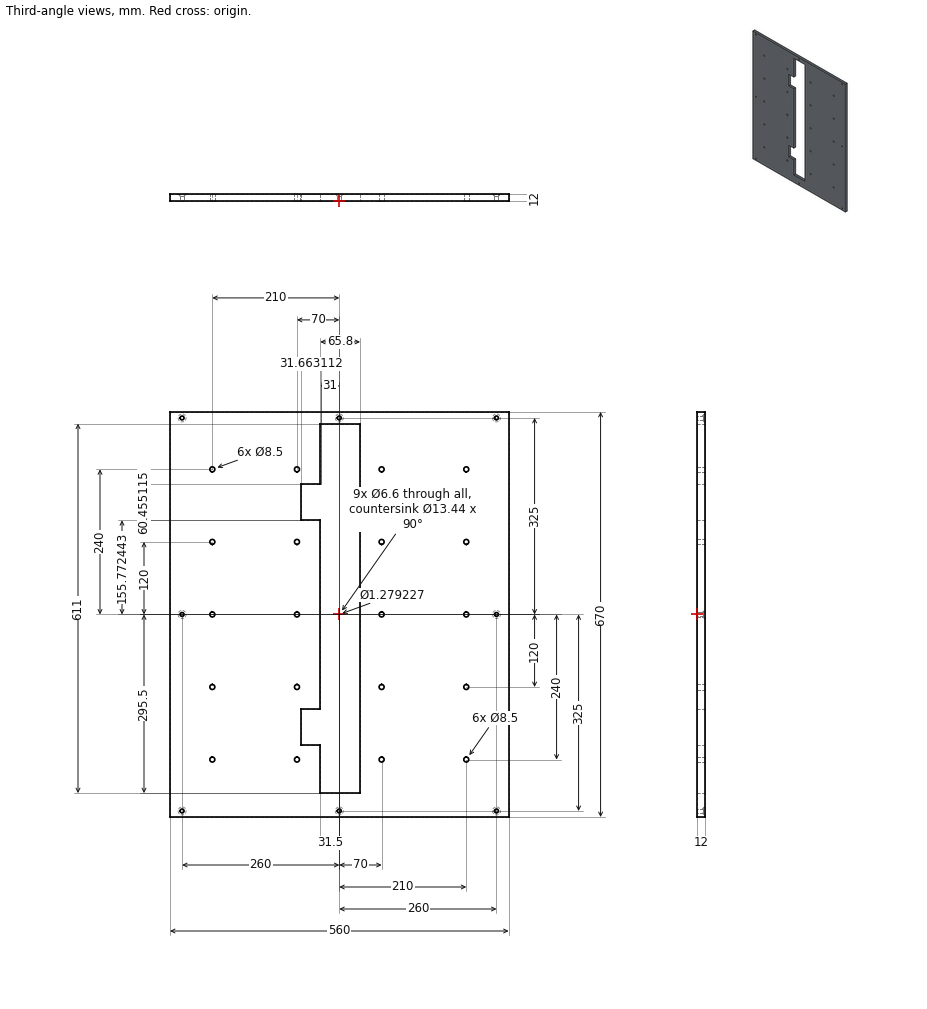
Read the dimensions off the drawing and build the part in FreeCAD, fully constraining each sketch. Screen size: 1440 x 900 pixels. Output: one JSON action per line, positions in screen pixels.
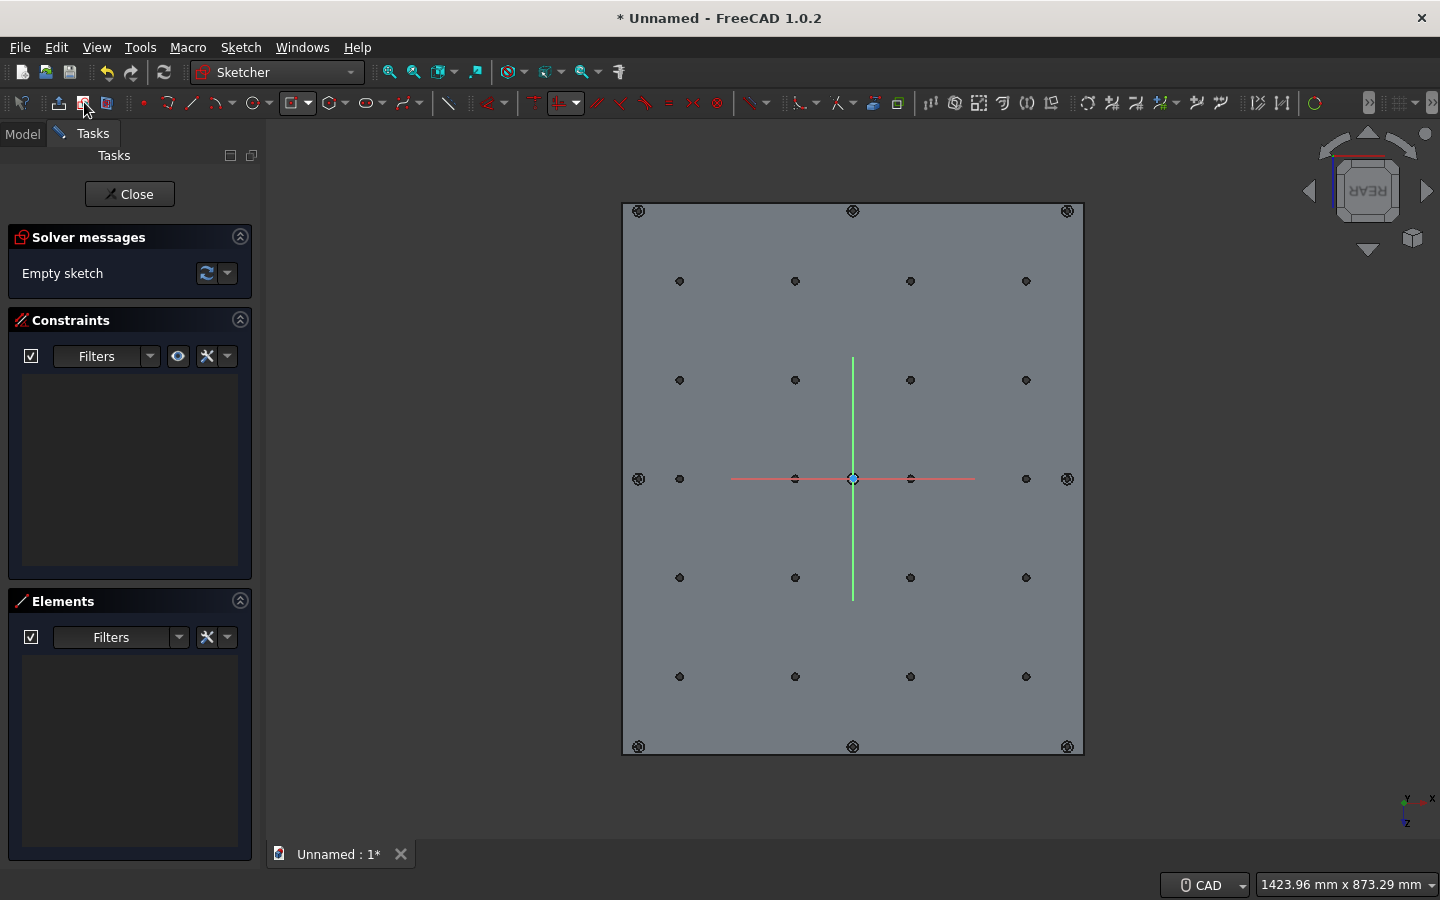
{"action": "left_click", "coordinate": [310, 104]}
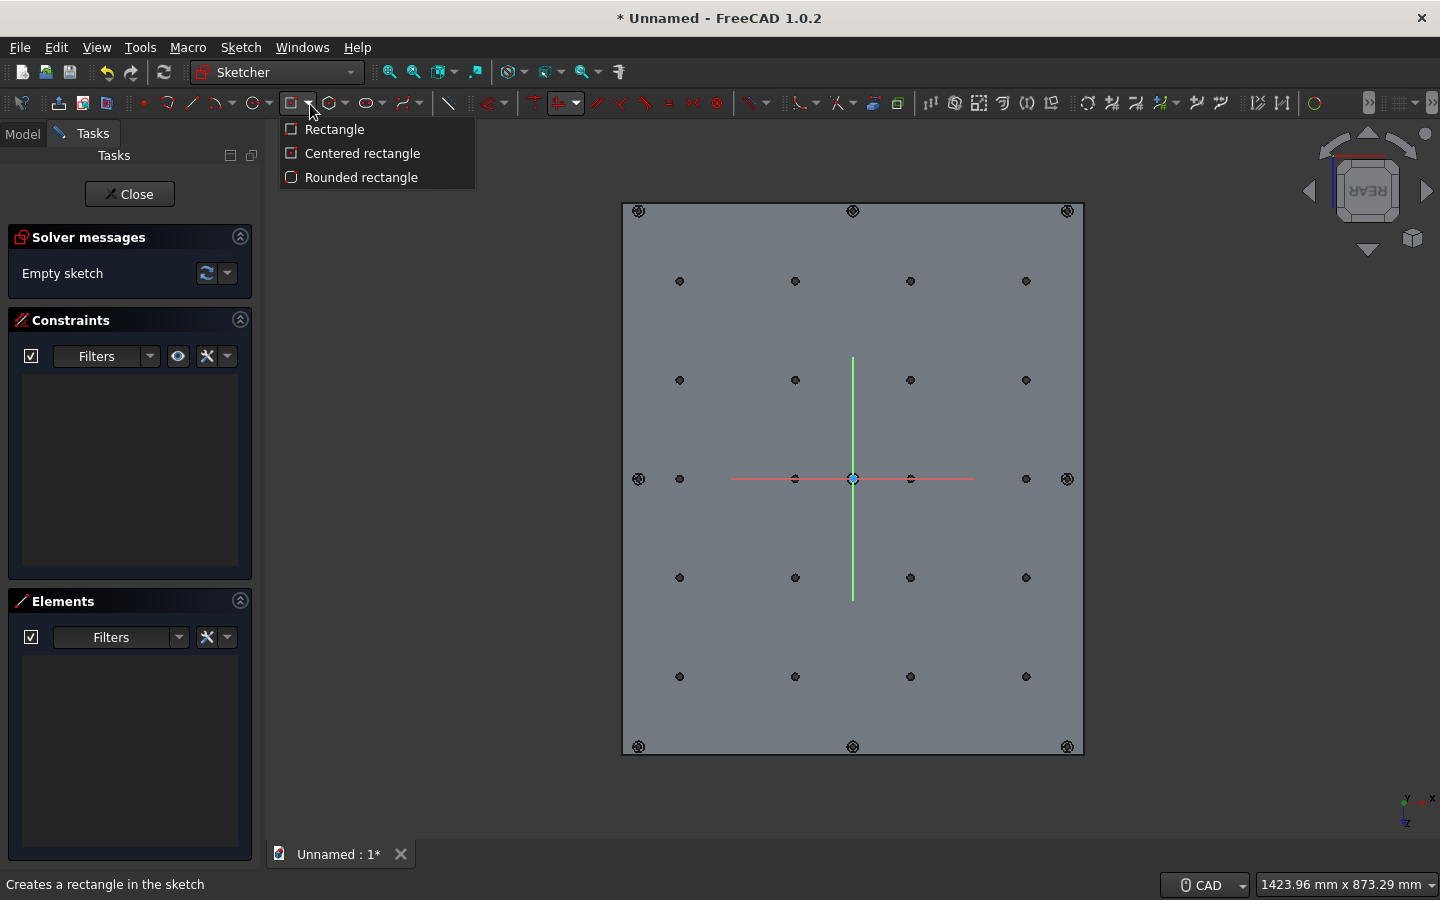
{"action": "left_click", "coordinate": [378, 129]}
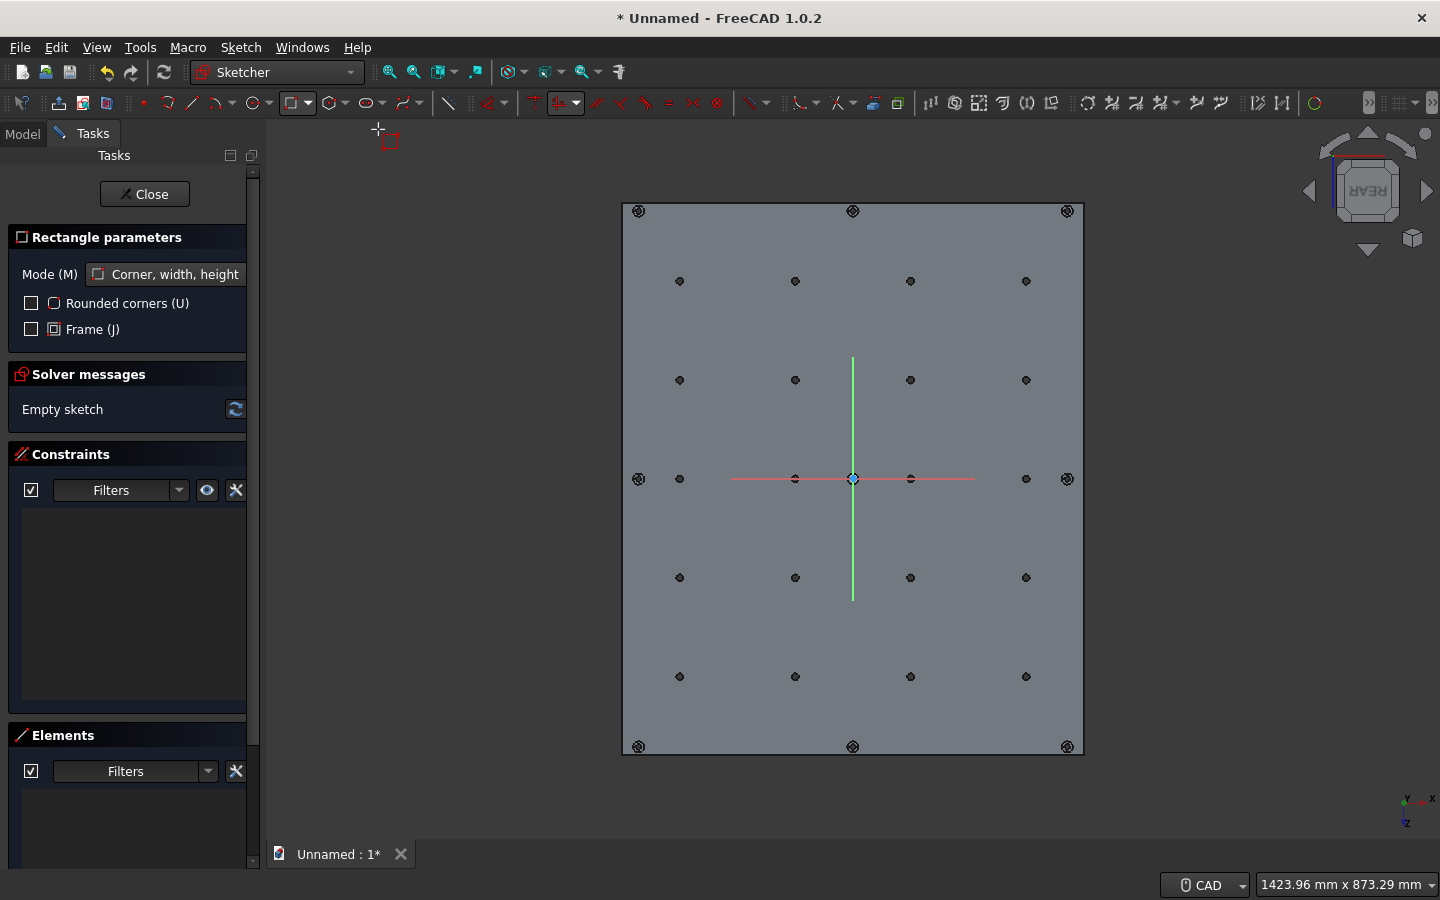
{"action": "left_click", "coordinate": [827, 235]}
{"action": "left_click", "coordinate": [881, 739]}
{"action": "key", "text": "Escape"}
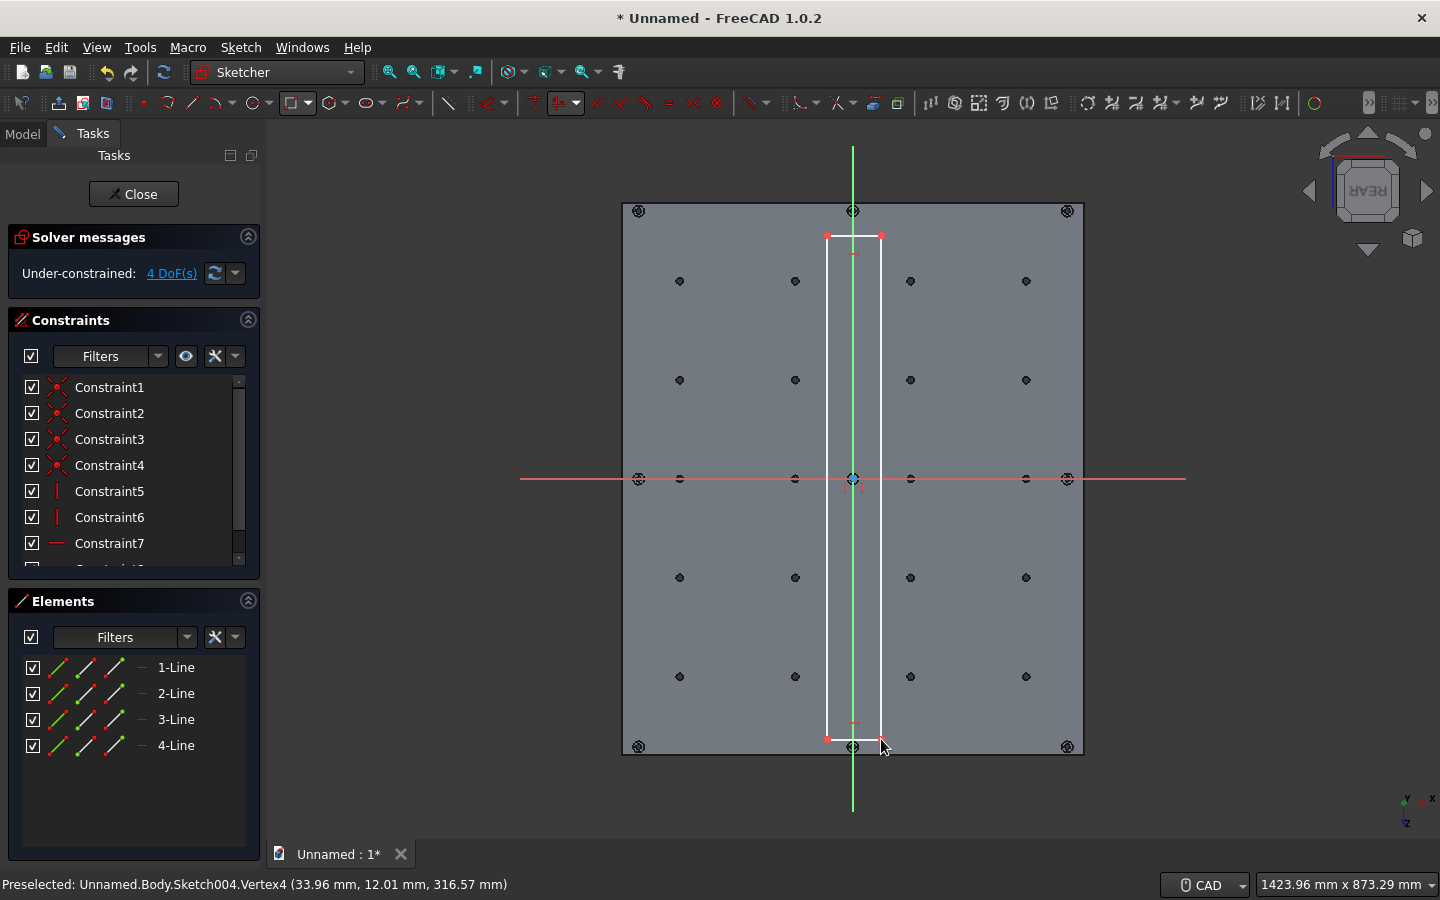
{"action": "left_click", "coordinate": [488, 104]}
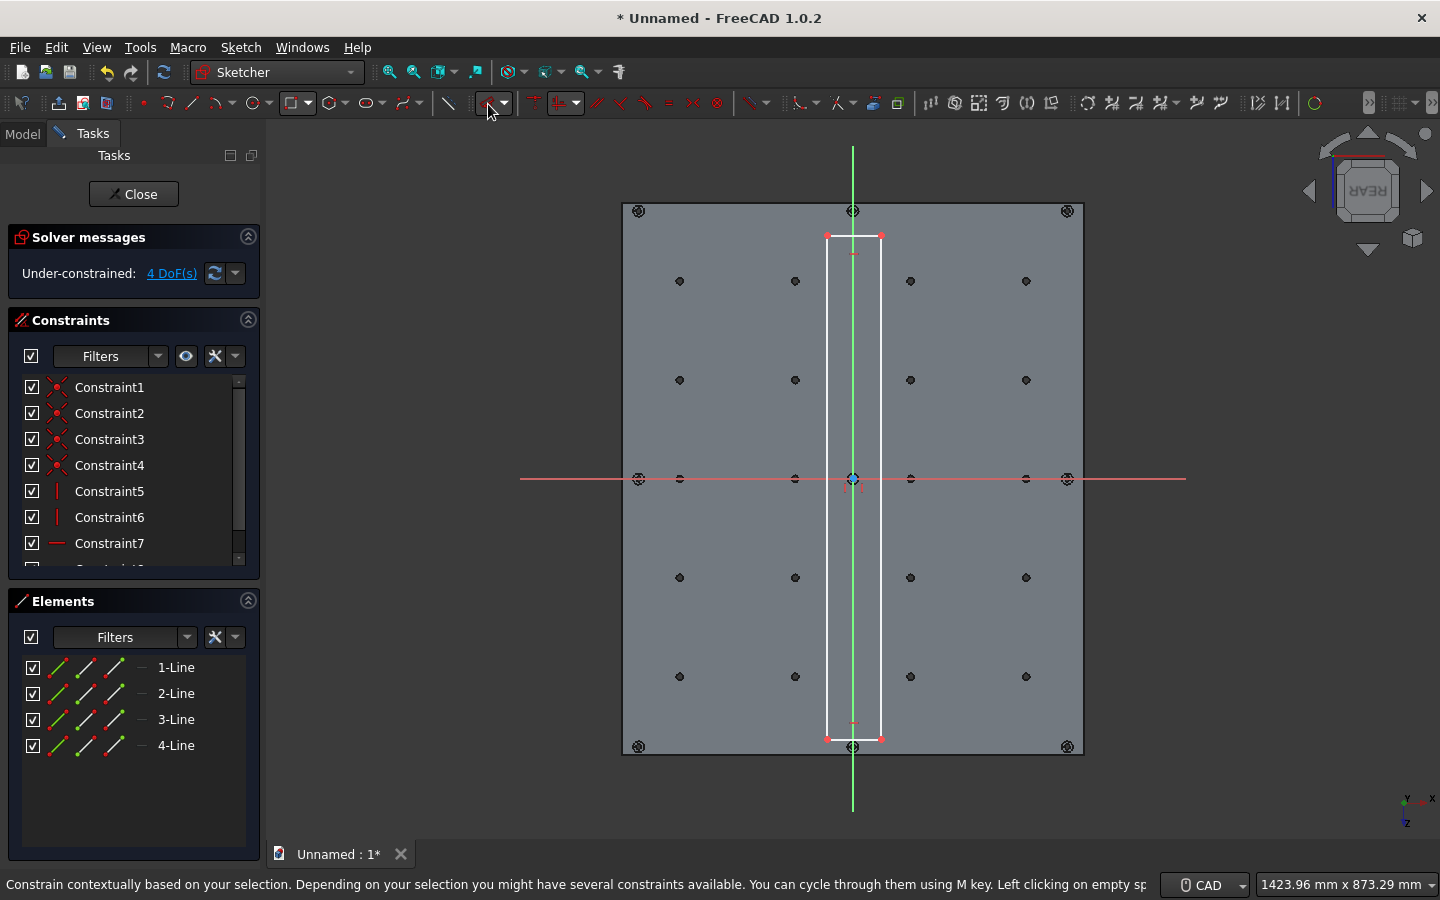
{"action": "left_click", "coordinate": [827, 387]}
{"action": "left_click", "coordinate": [793, 372]}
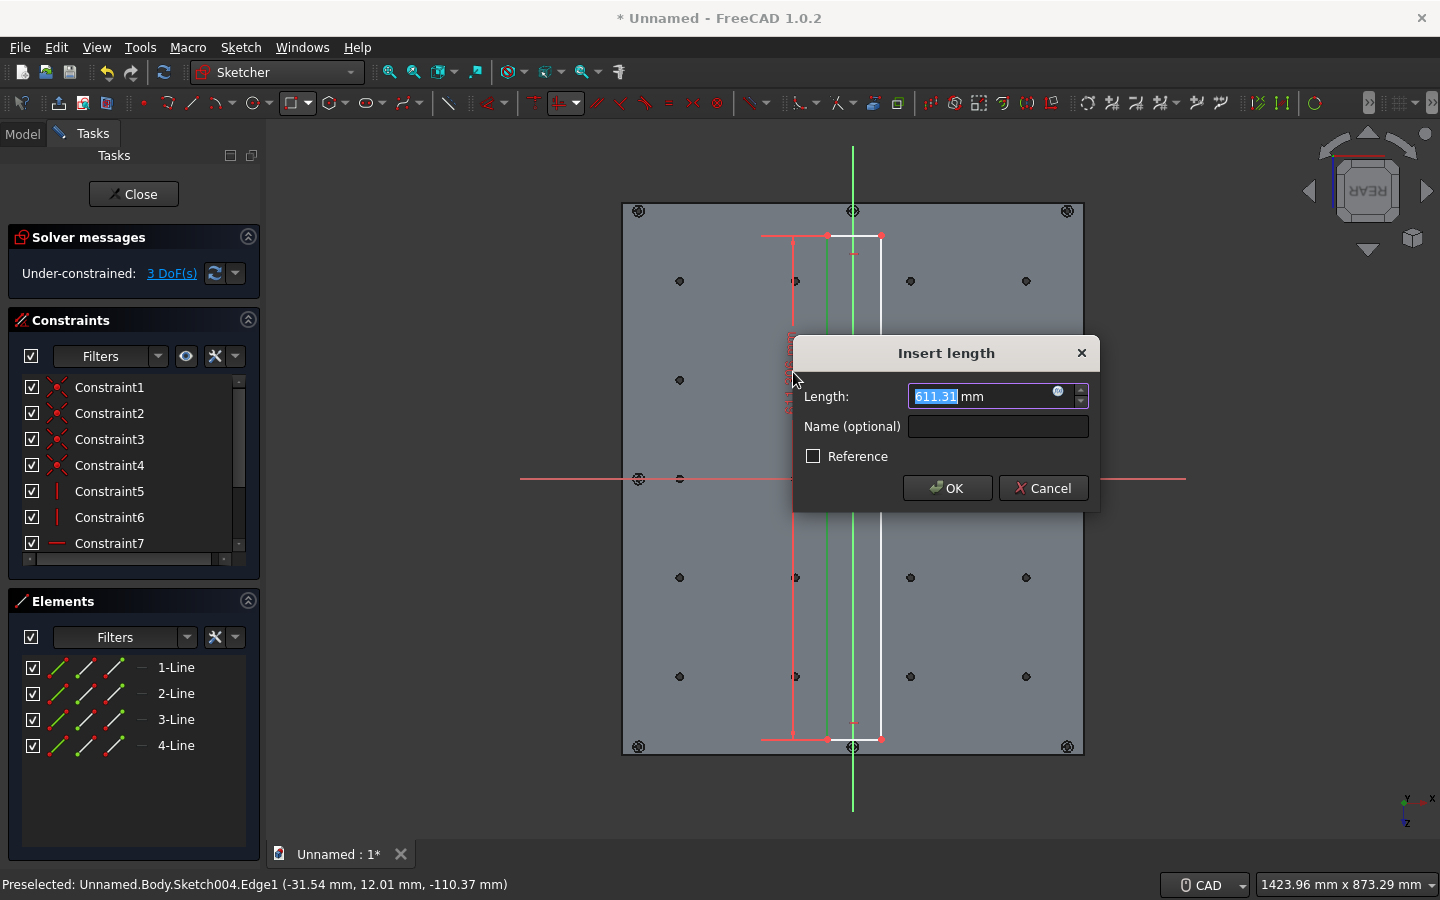
{"action": "type", "text": "611"}
{"action": "key", "text": "Return"}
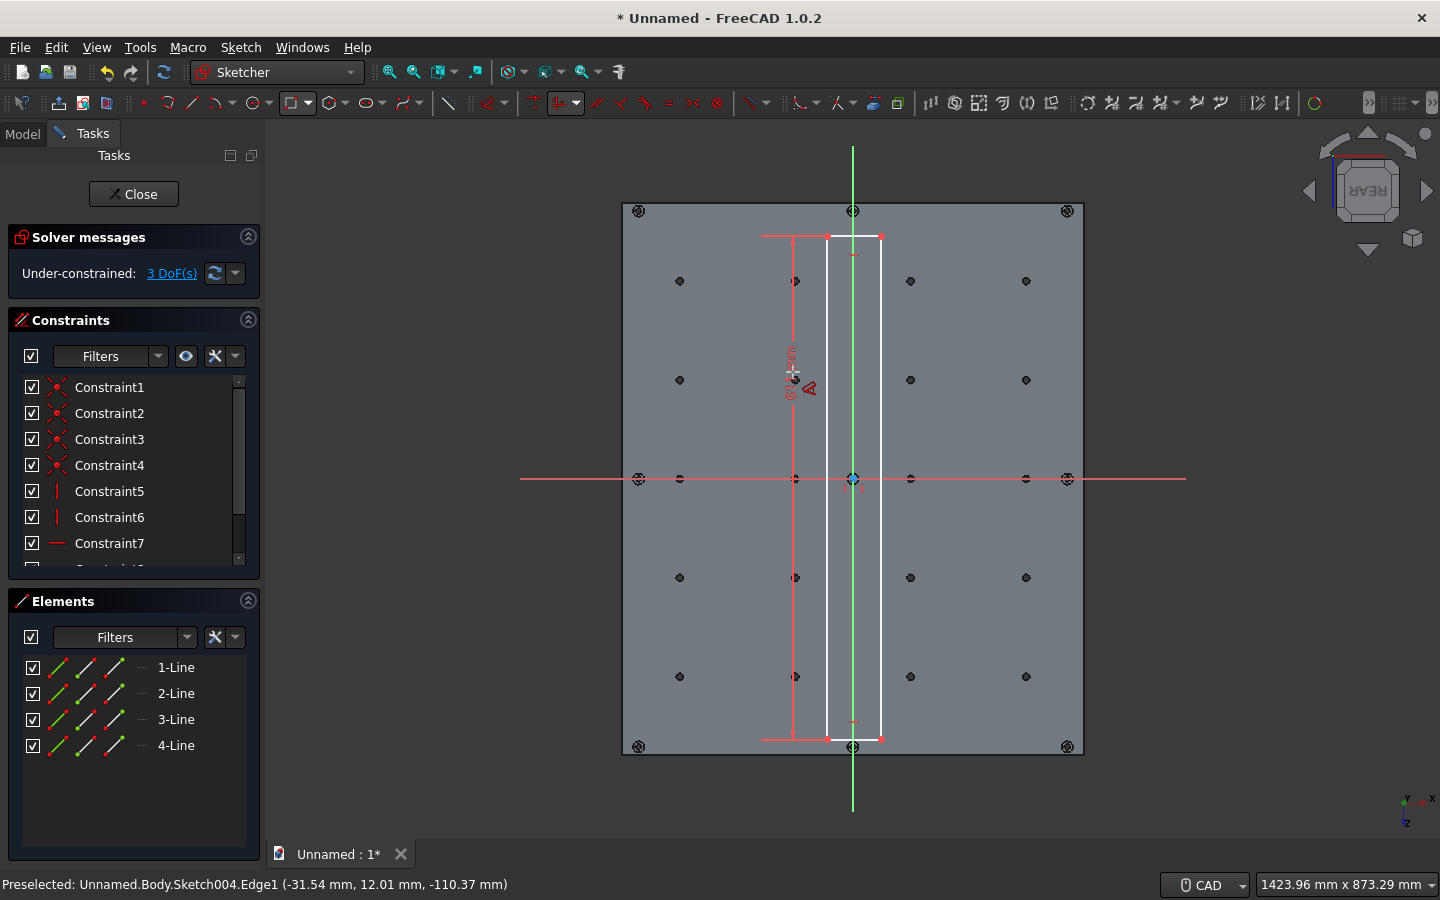
{"action": "scroll", "coordinate": [843, 740], "scroll_direction": "up", "scroll_amount": 2}